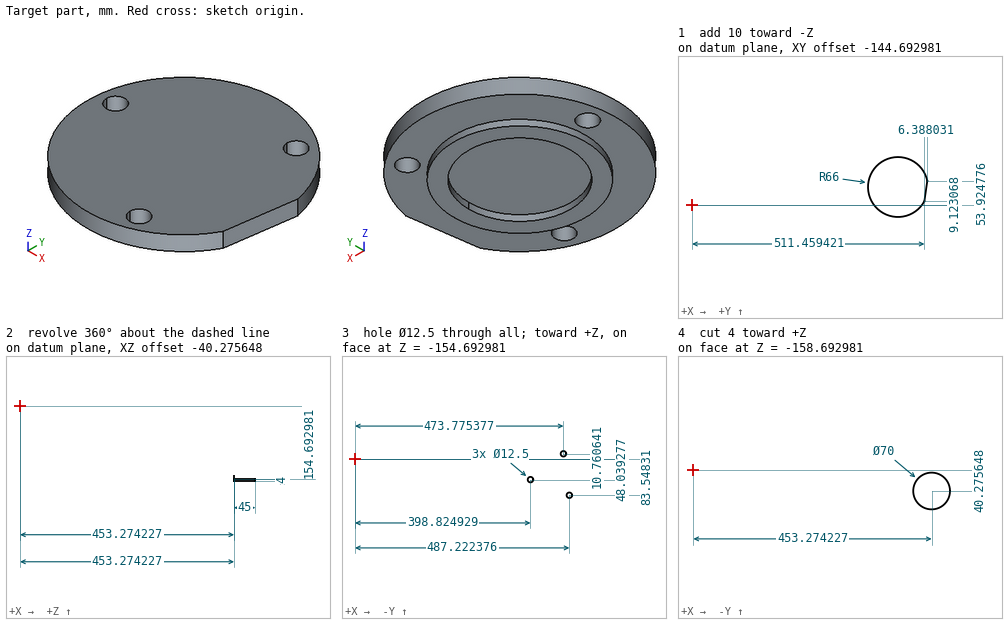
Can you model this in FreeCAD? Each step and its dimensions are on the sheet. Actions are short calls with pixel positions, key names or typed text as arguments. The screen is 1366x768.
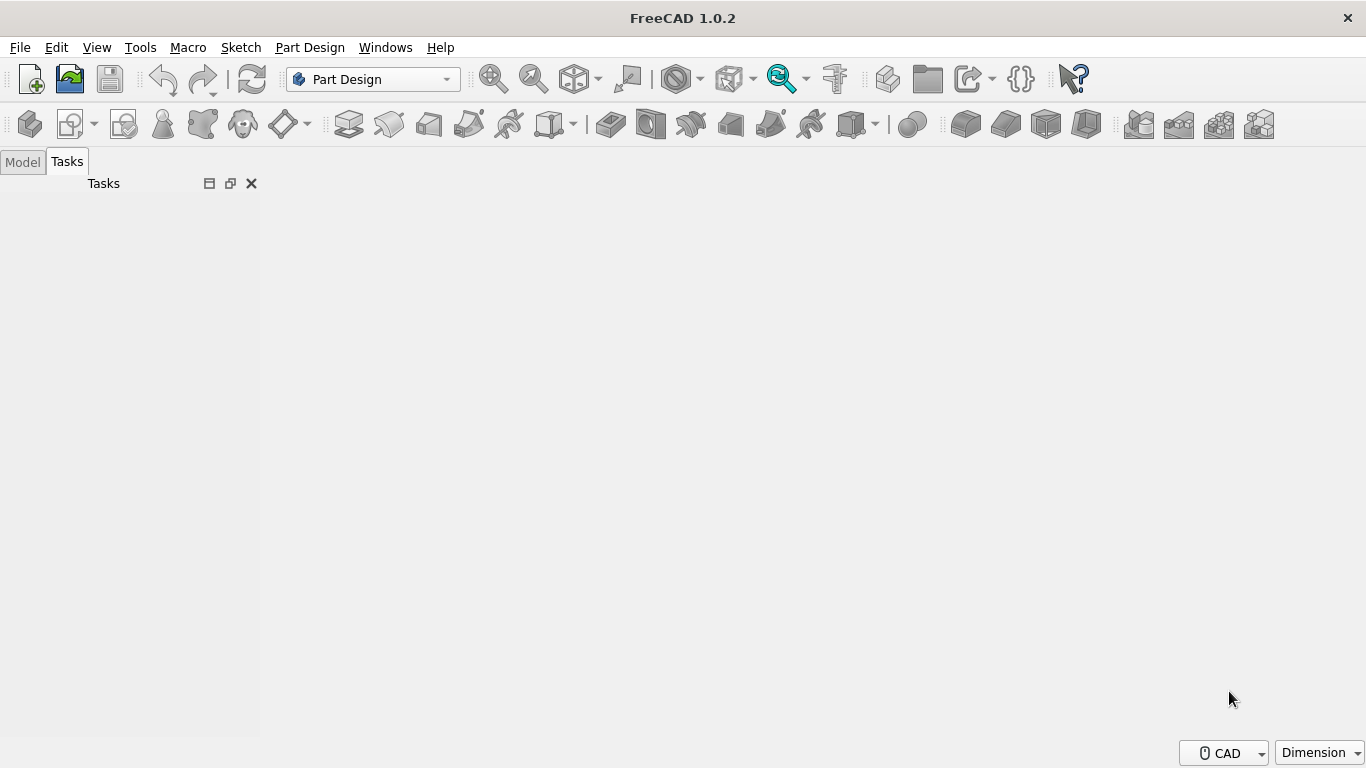
key(ctrl+n)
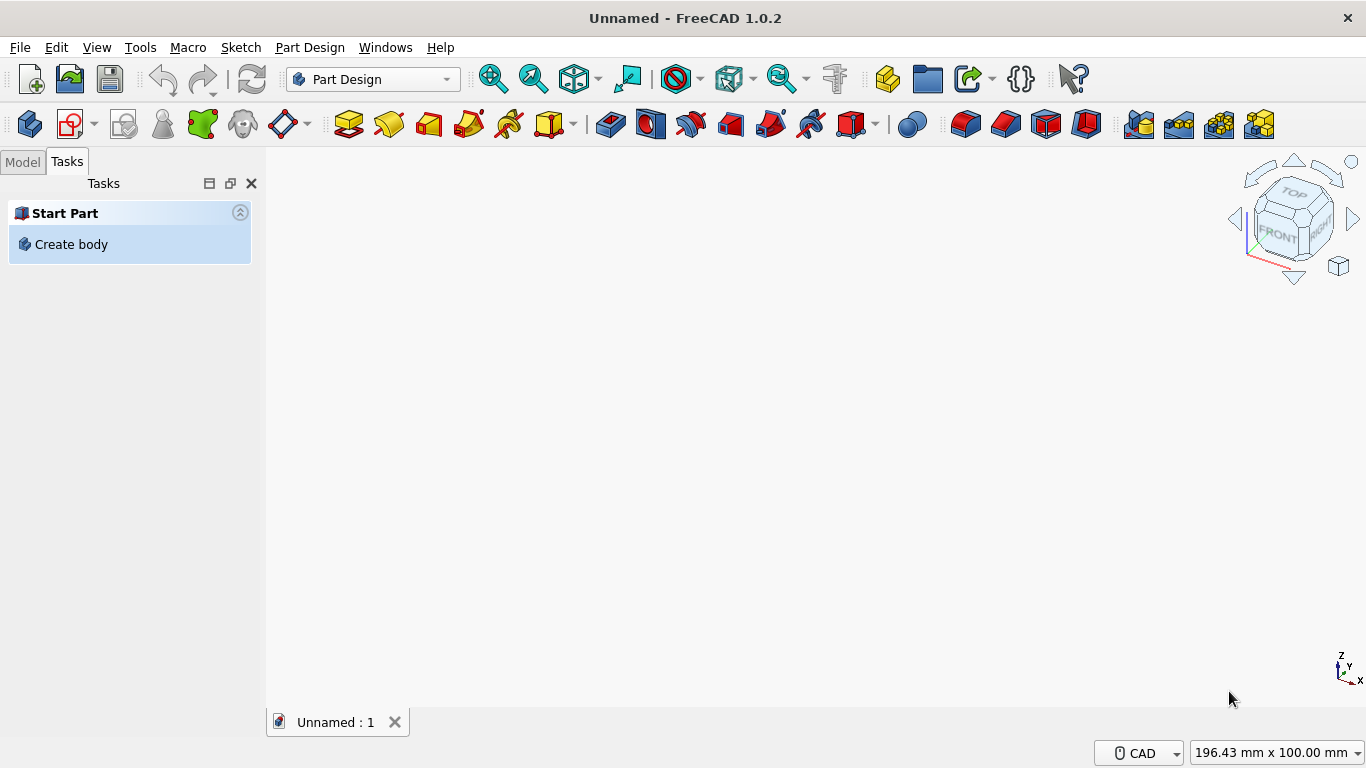
click(30, 124)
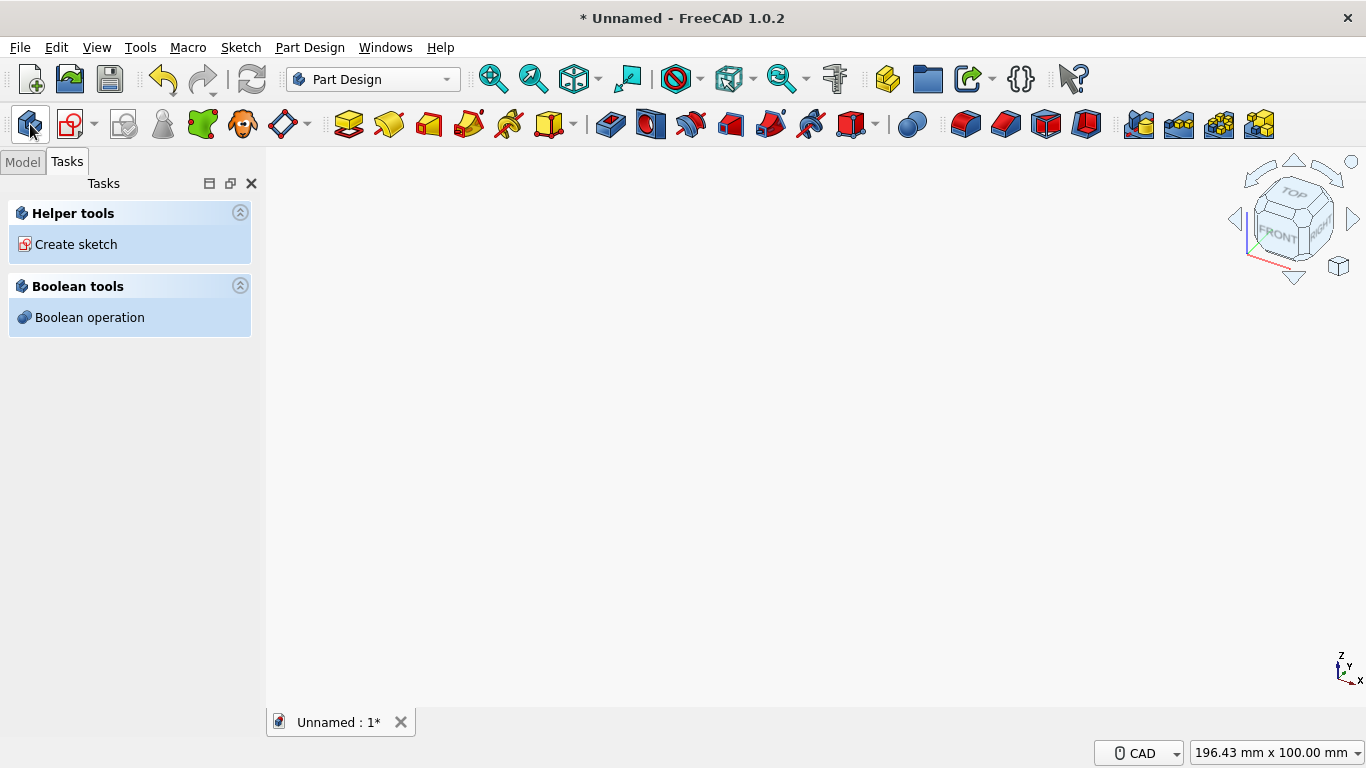
click(23, 161)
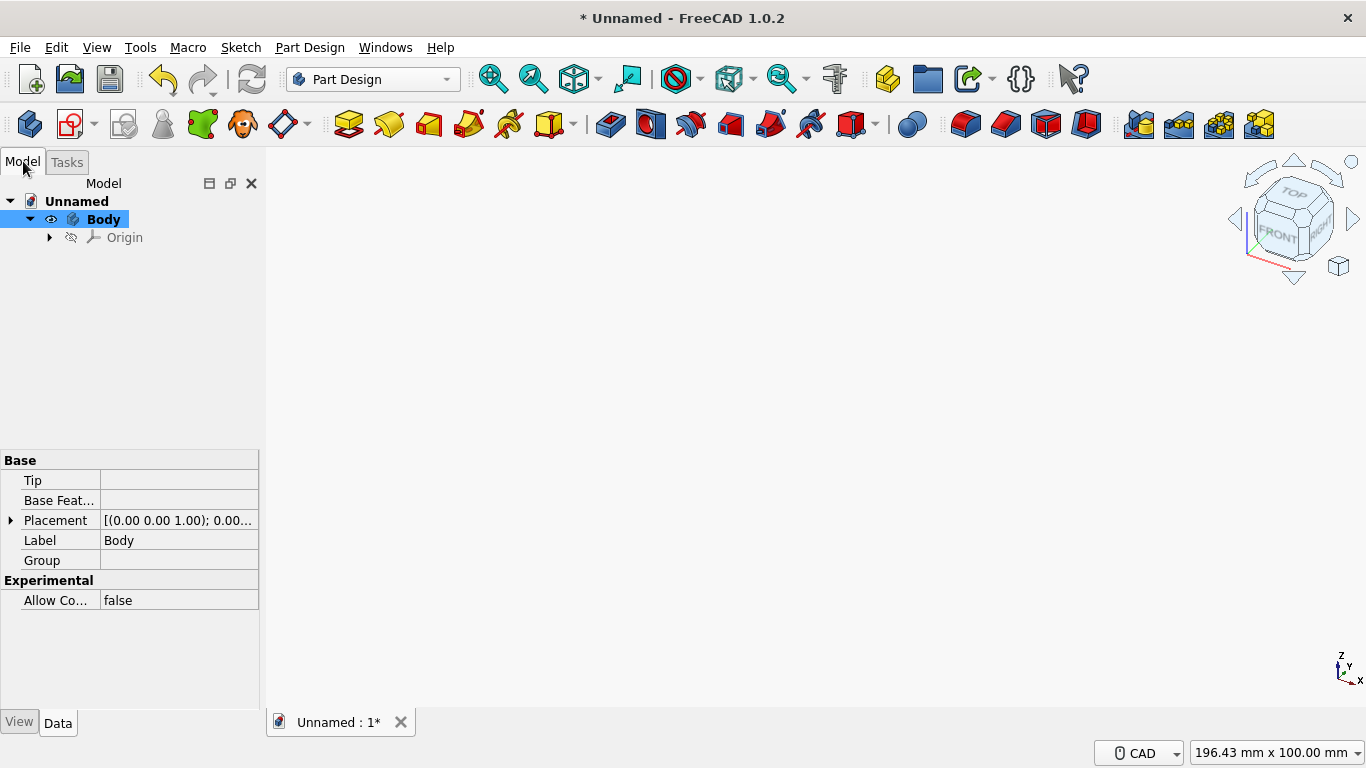
click(50, 237)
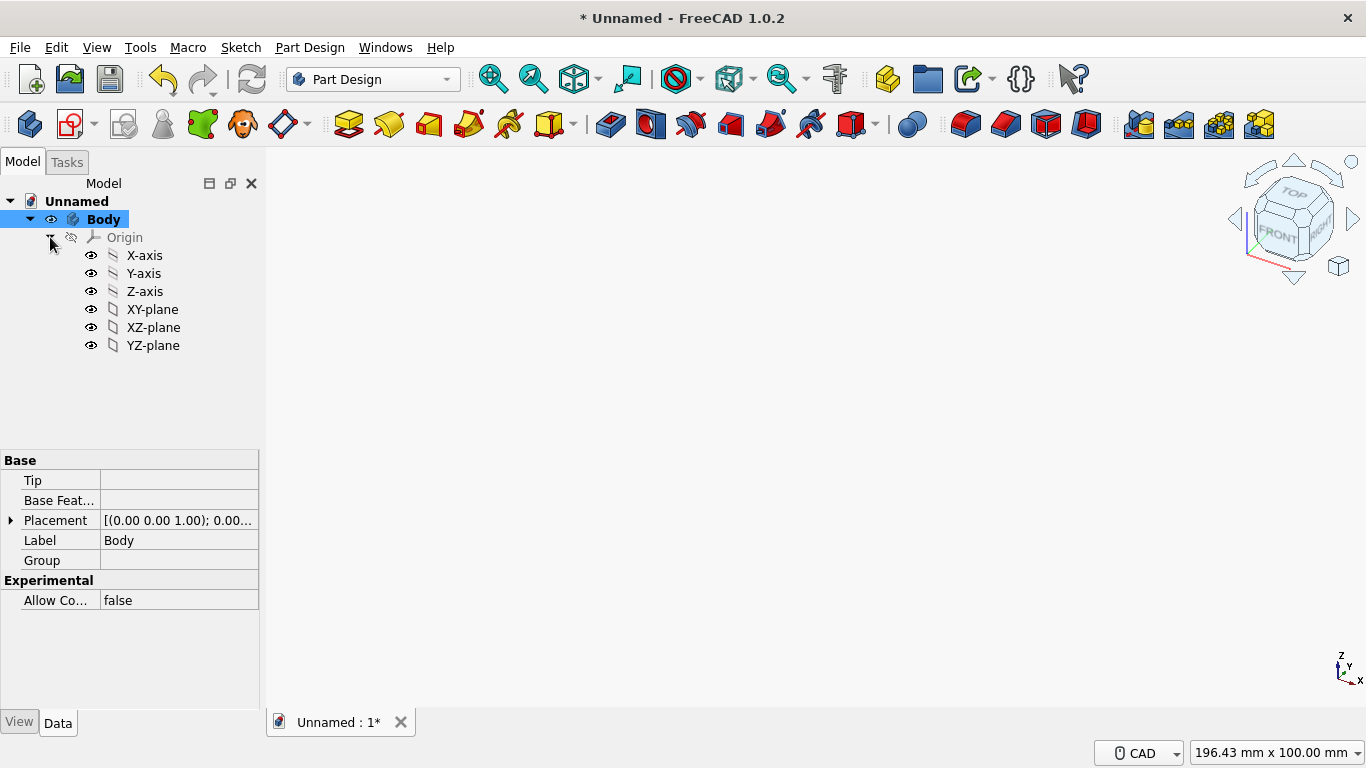
click(136, 309)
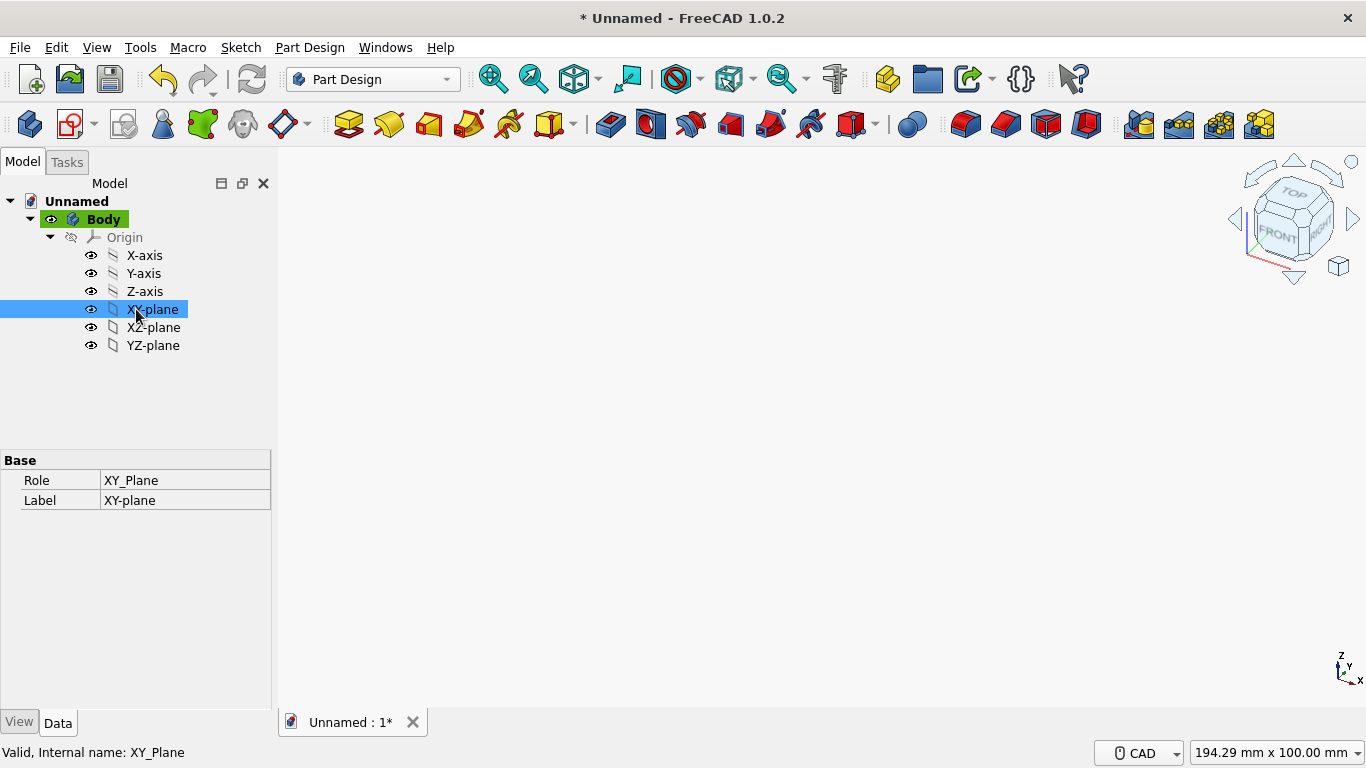
click(284, 124)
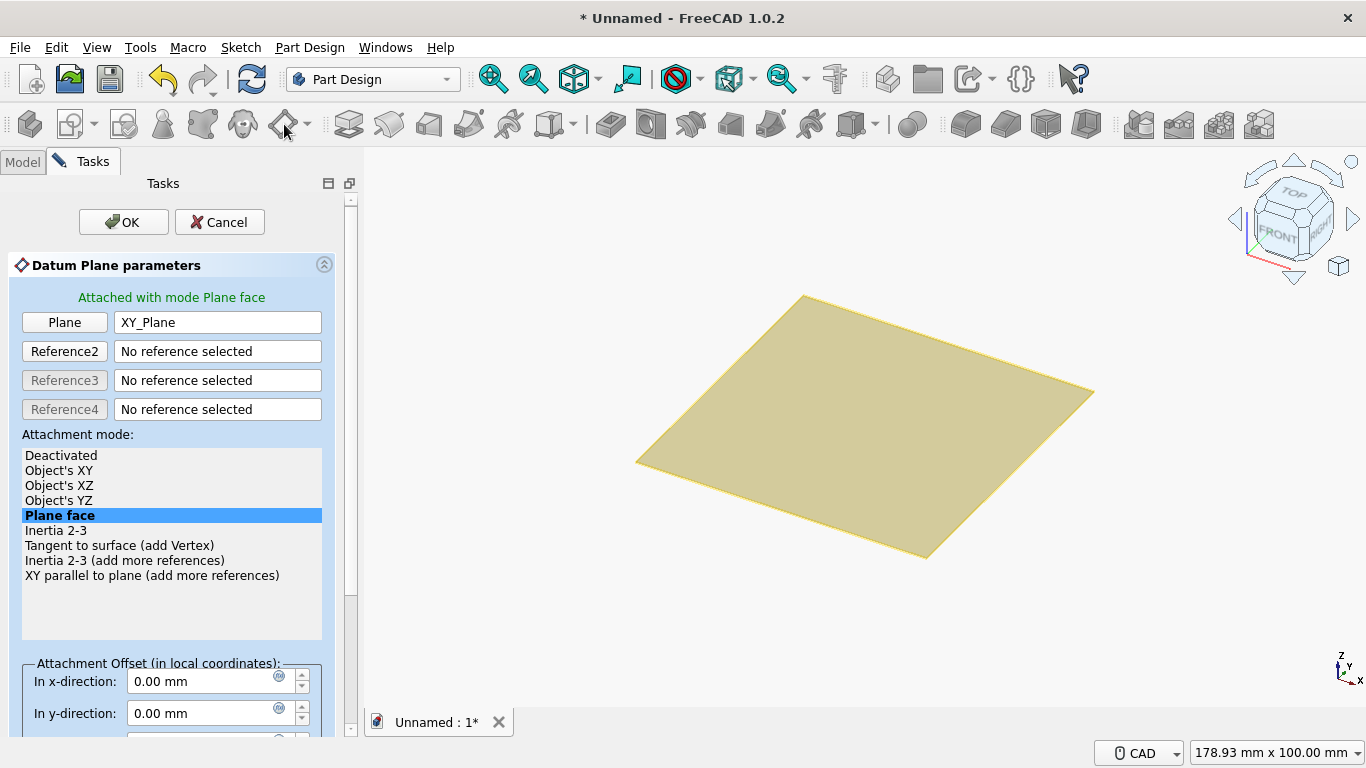
scroll(351, 464, down, 2)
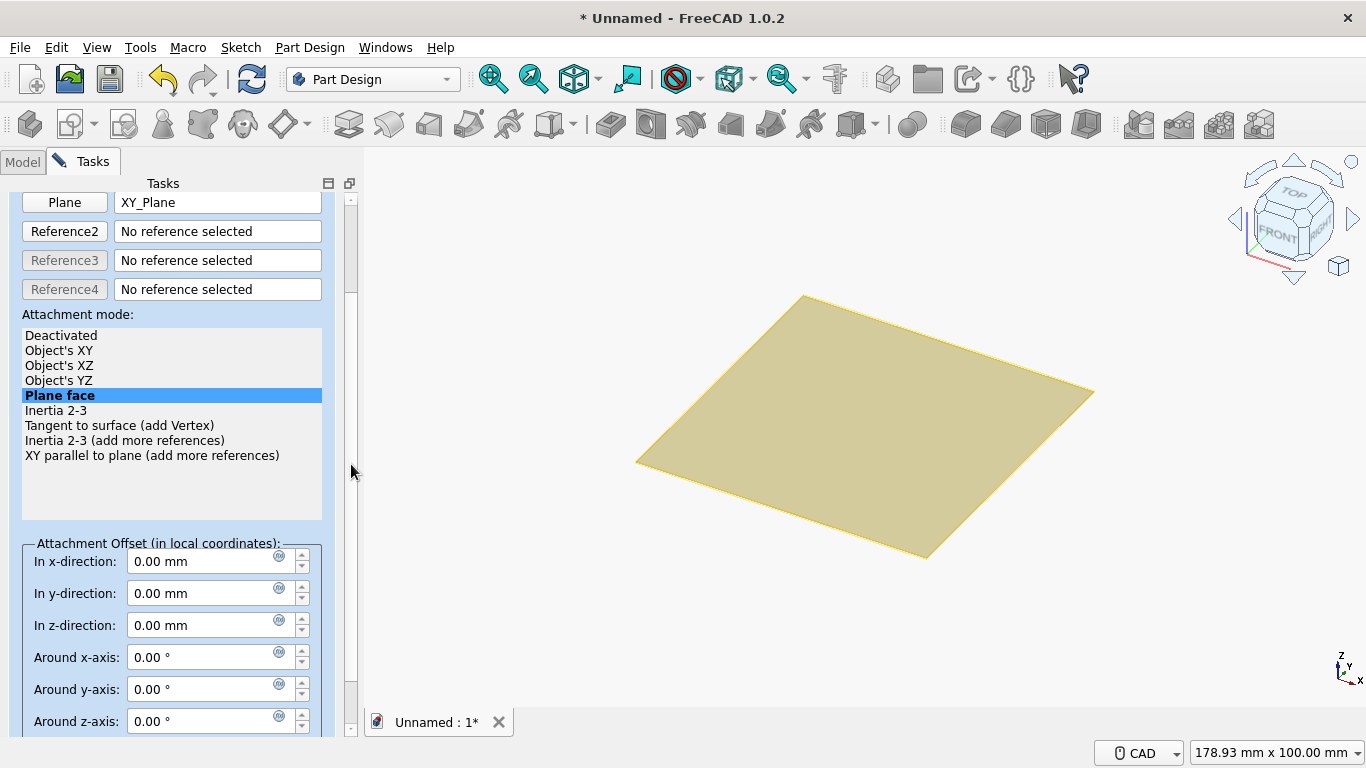
triple_click(210, 625)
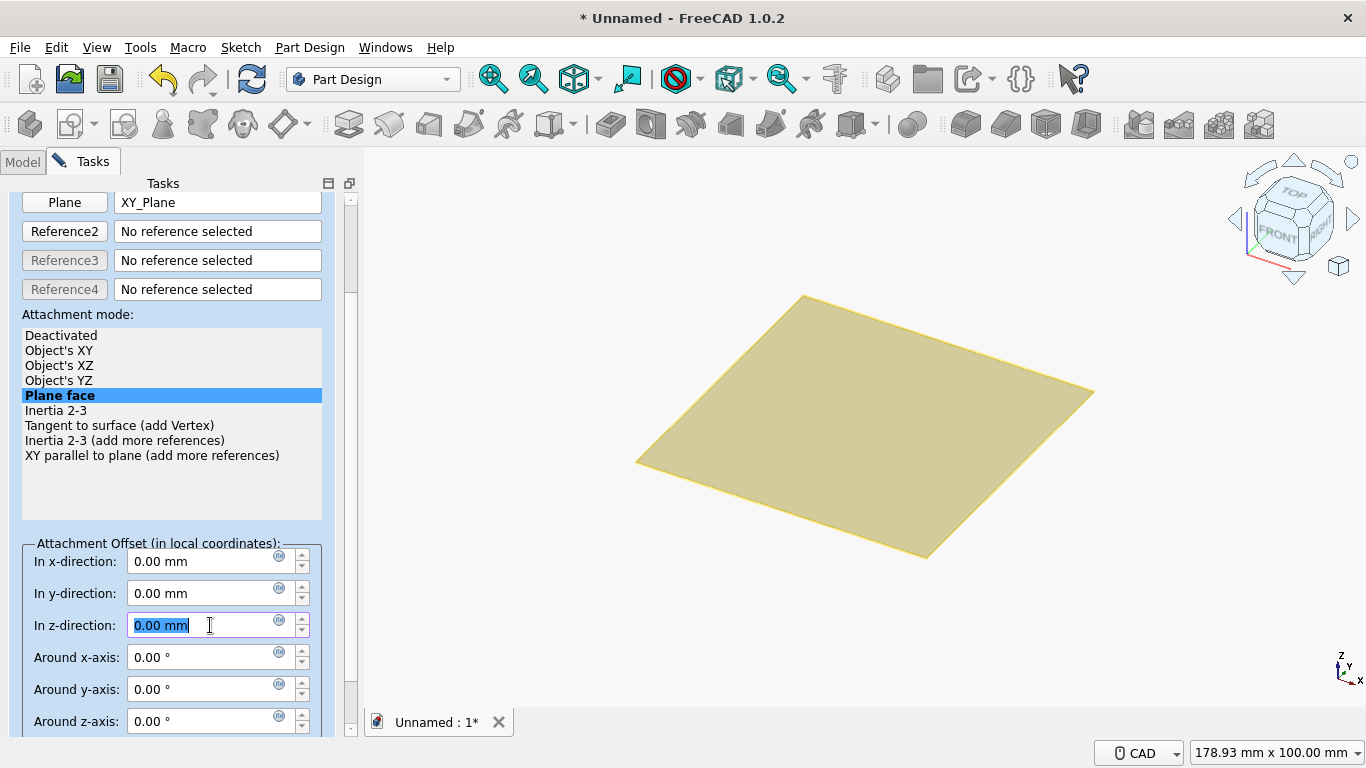
text(-144.692981)
key(Tab)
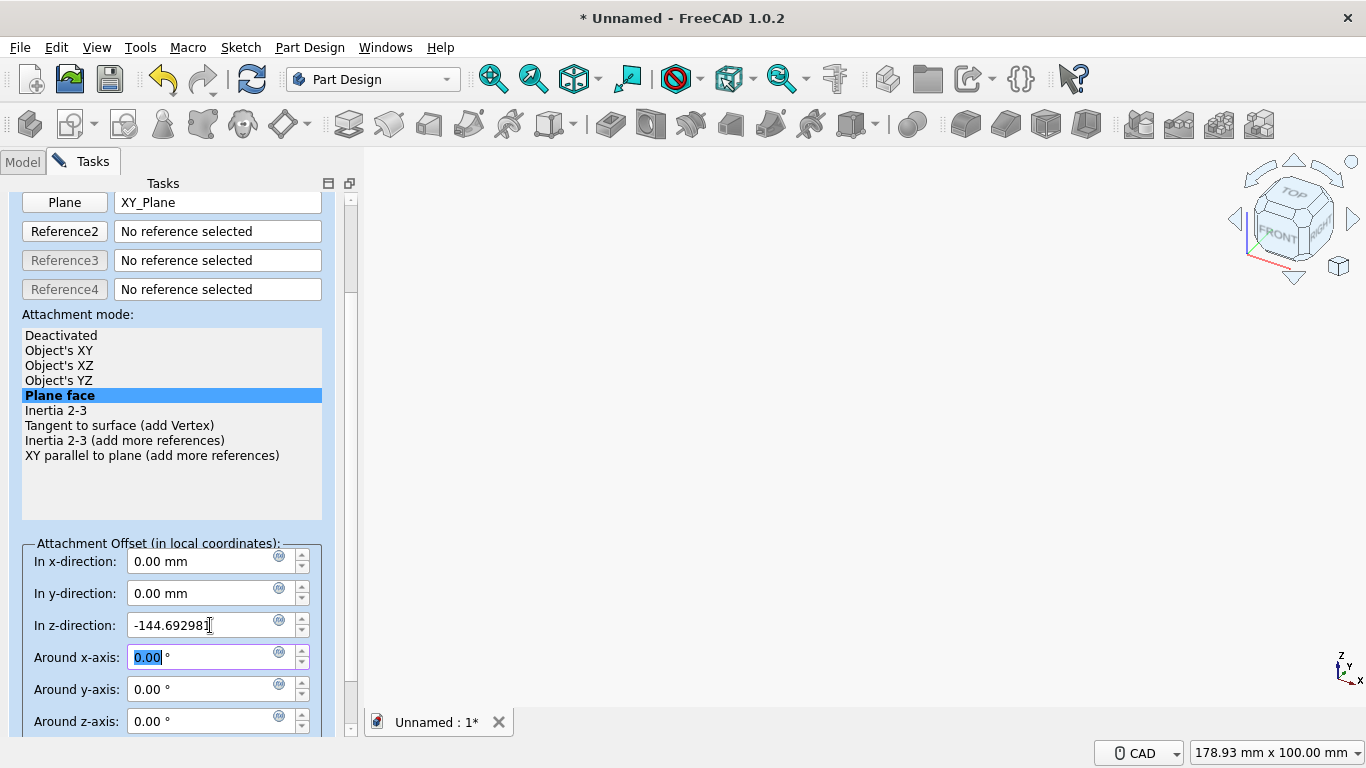
scroll(351, 464, up, 3)